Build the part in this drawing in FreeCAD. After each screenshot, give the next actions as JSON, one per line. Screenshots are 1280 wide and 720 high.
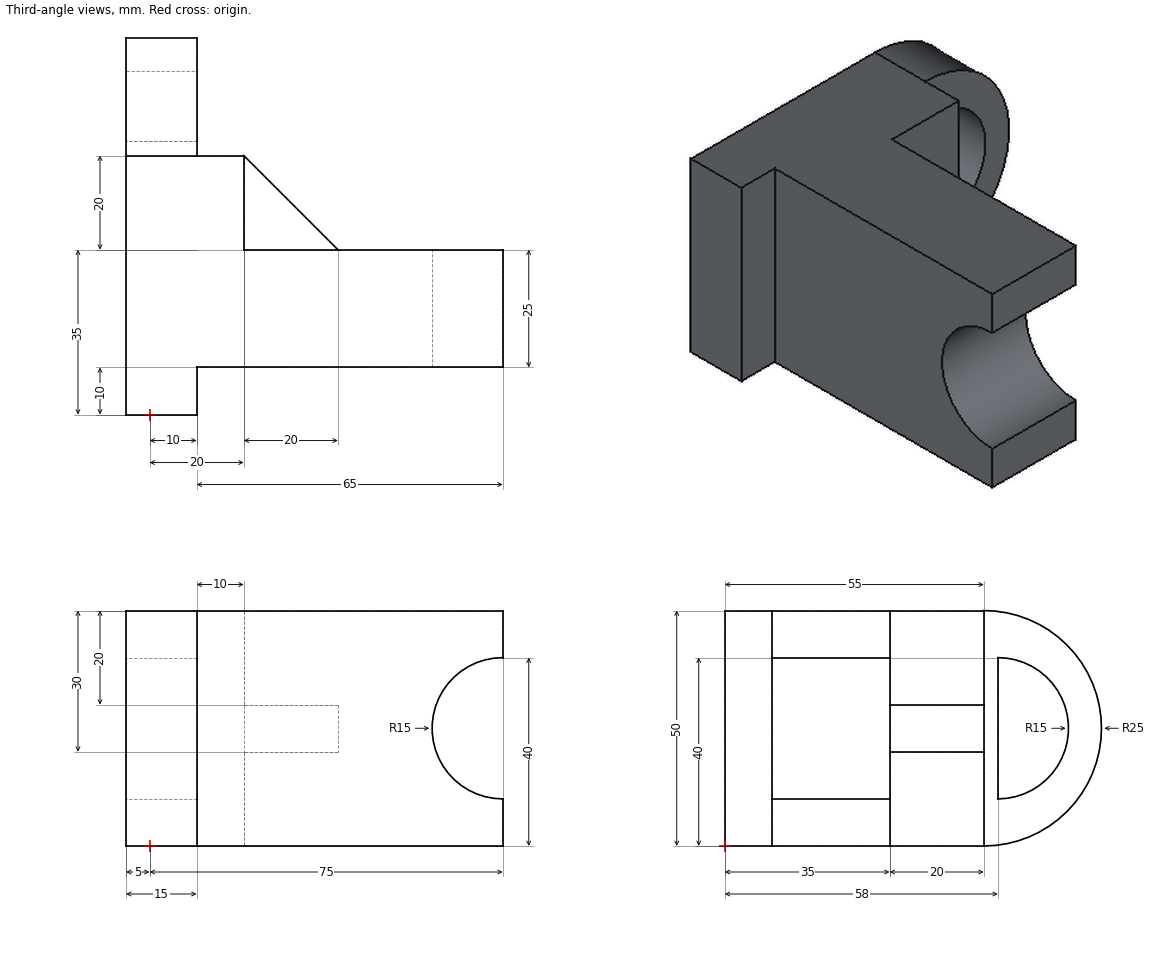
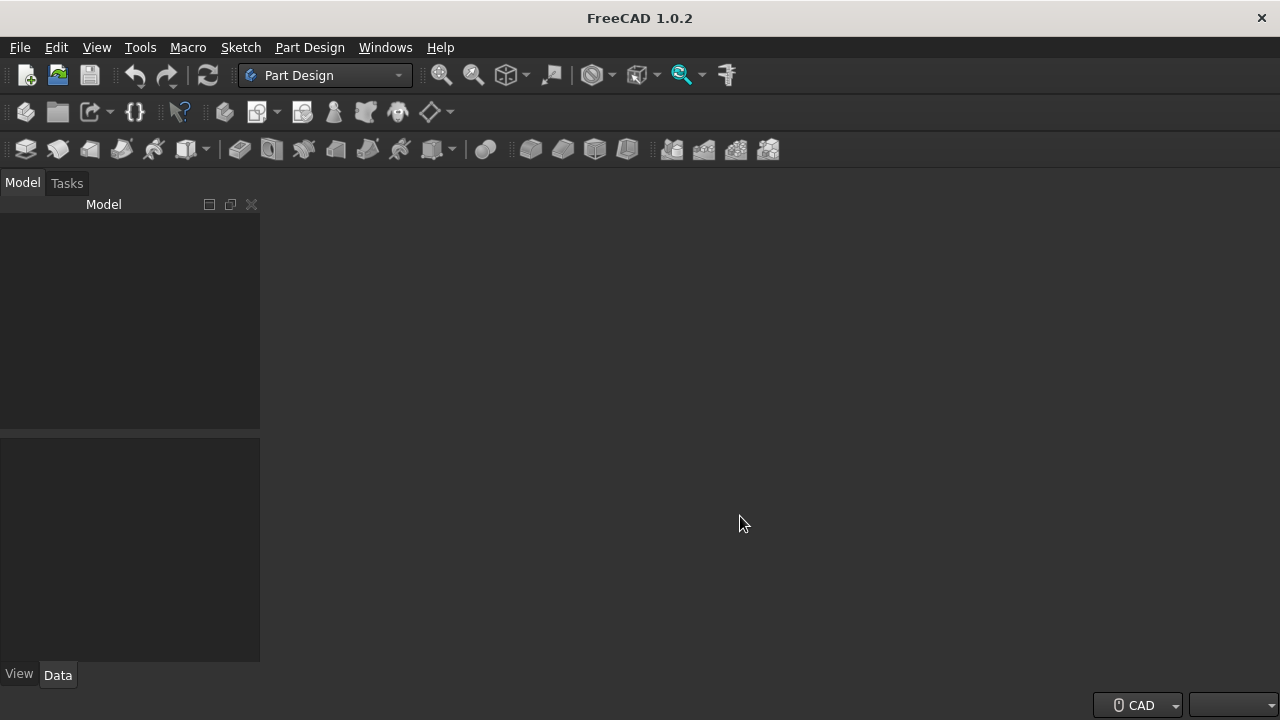
{"action": "left_click", "coordinate": [26, 76]}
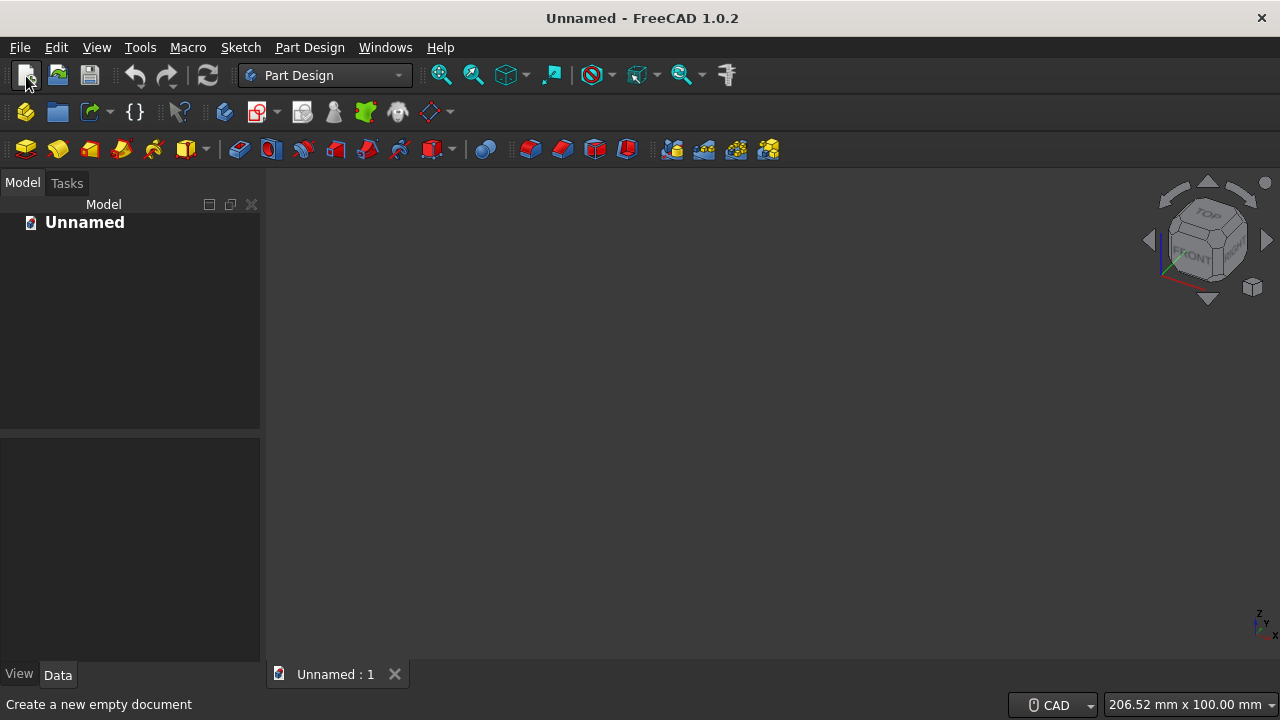
{"action": "left_click", "coordinate": [258, 112]}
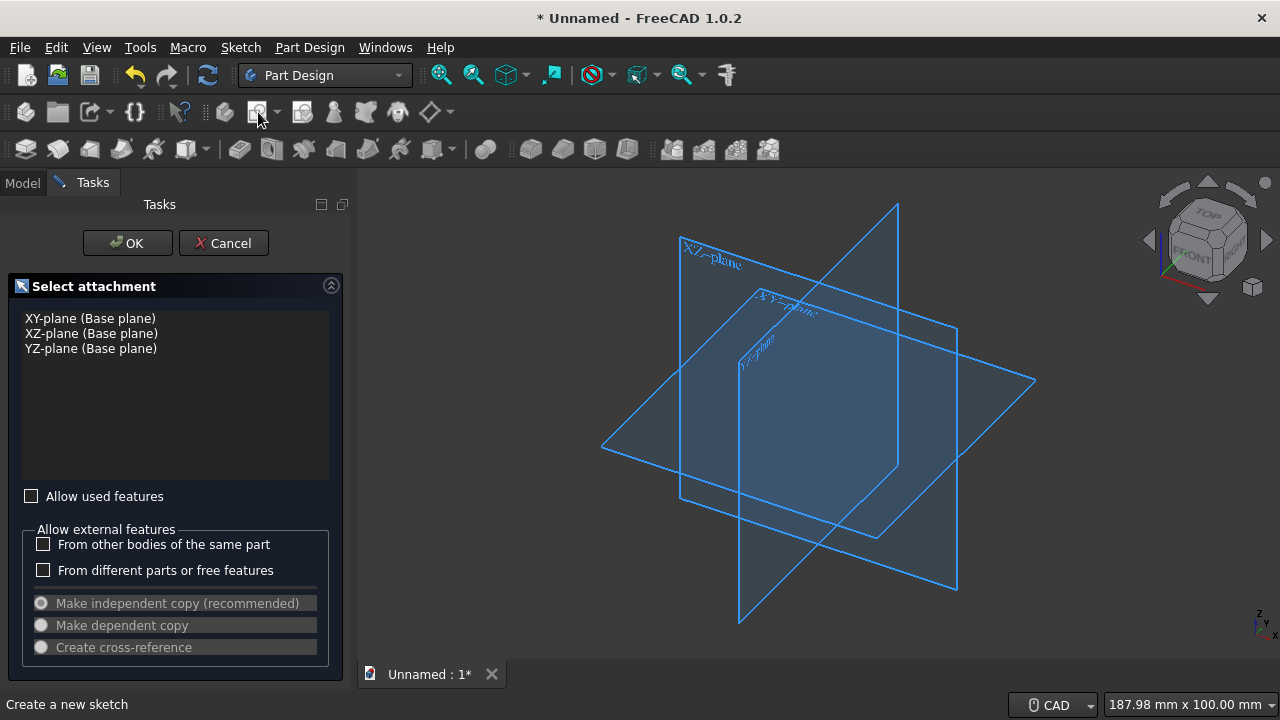
{"action": "left_click", "coordinate": [82, 318]}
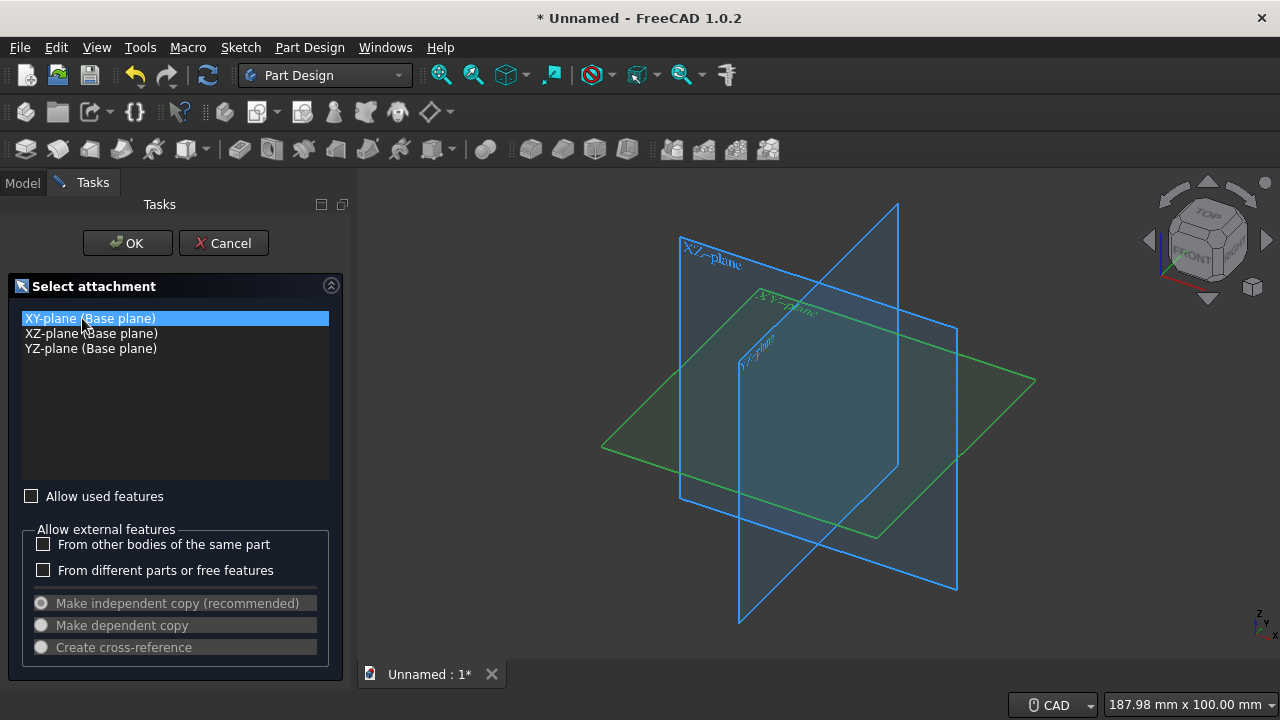
{"action": "left_click", "coordinate": [128, 243]}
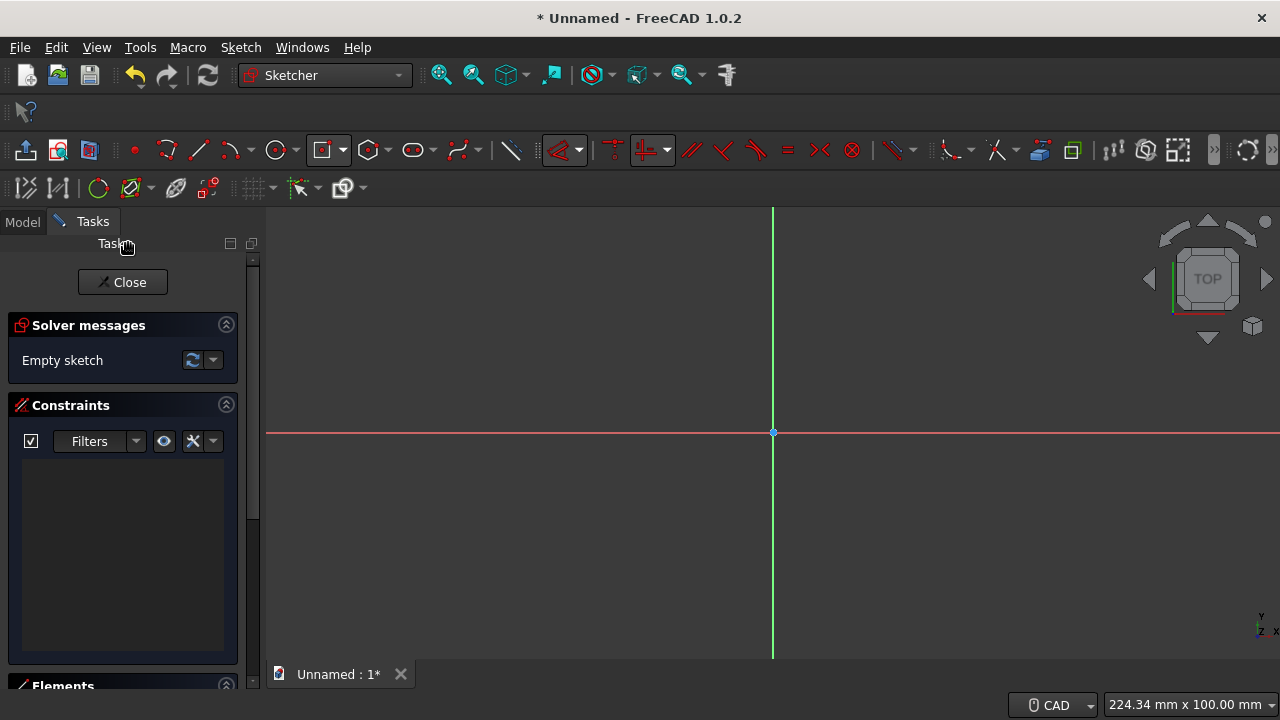
{"action": "scroll", "coordinate": [294, 631], "scroll_direction": "down", "scroll_amount": 1}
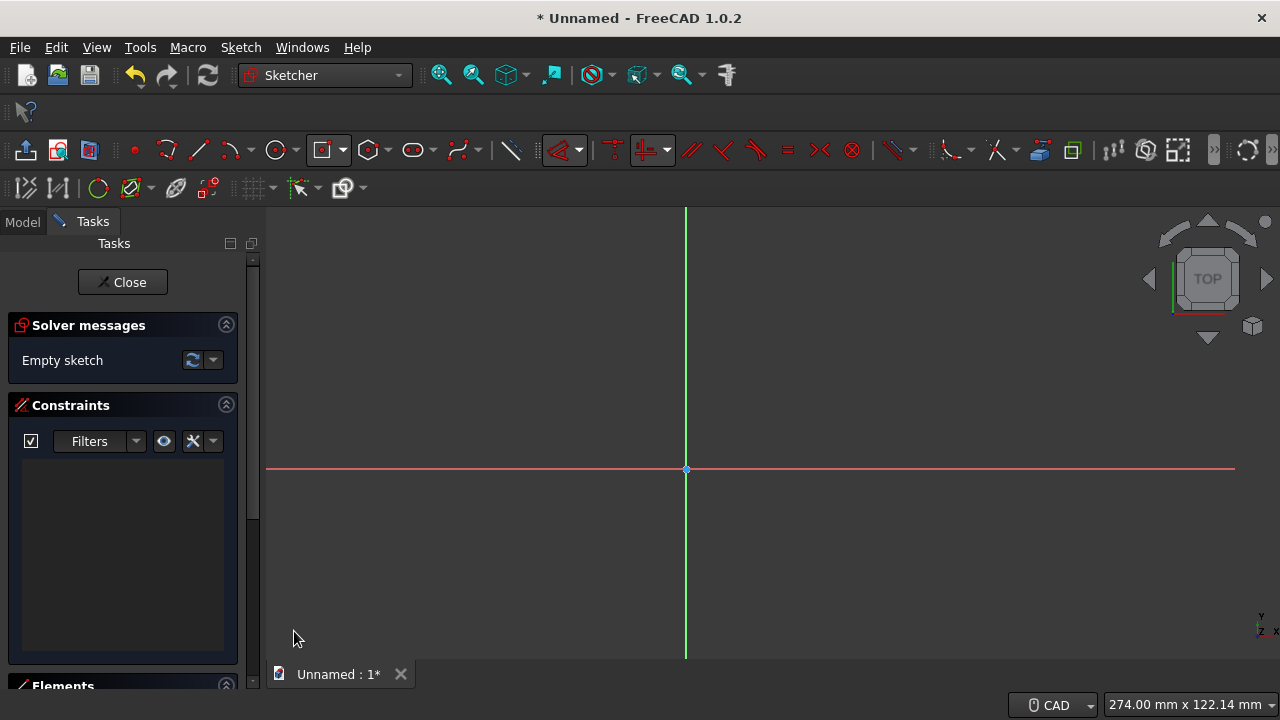
{"action": "scroll", "coordinate": [1070, 235], "scroll_direction": "up", "scroll_amount": 2}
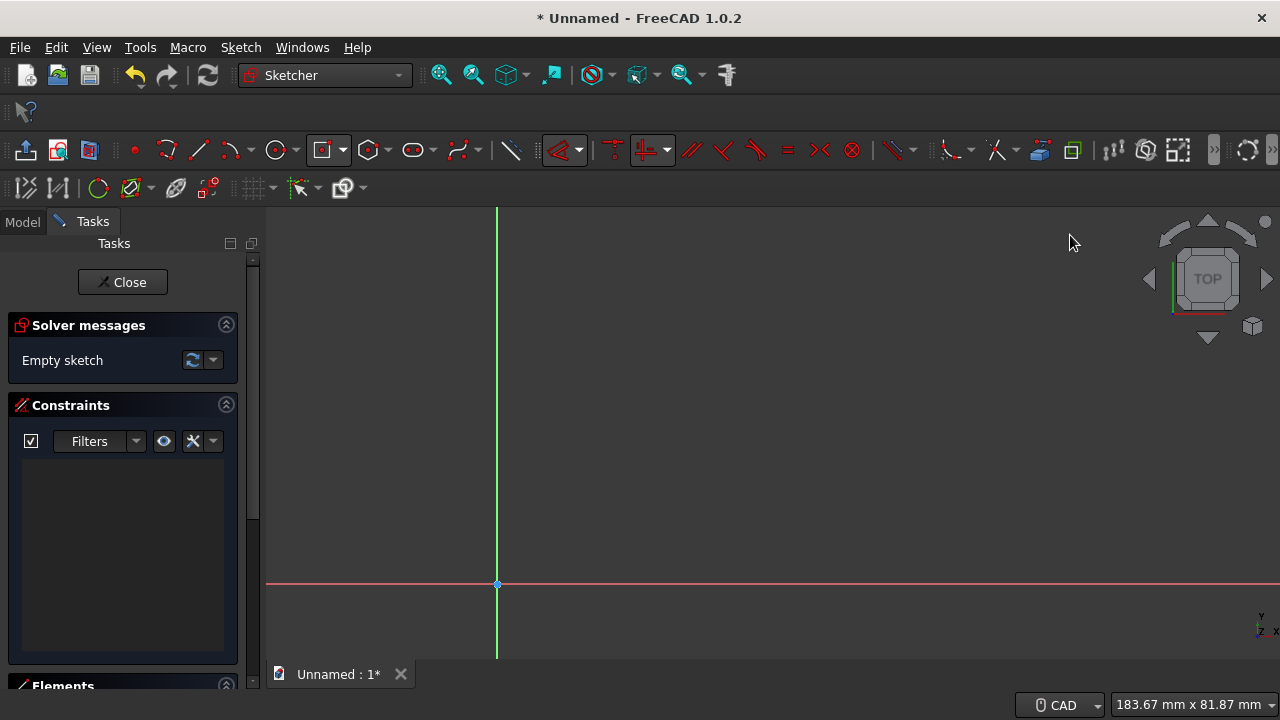
{"action": "left_click", "coordinate": [168, 150]}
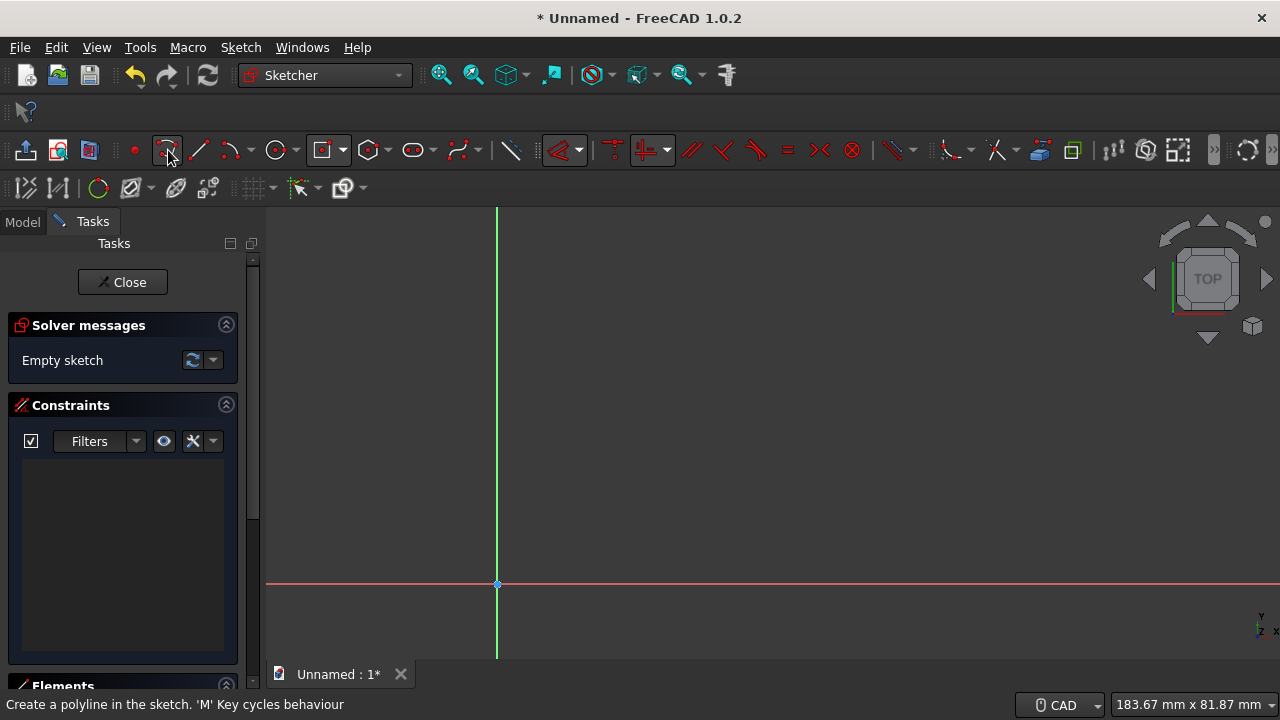
{"action": "left_click", "coordinate": [497, 584]}
{"action": "left_click", "coordinate": [552, 575]}
{"action": "left_click", "coordinate": [552, 529]}
{"action": "left_click", "coordinate": [911, 529]}
{"action": "left_click", "coordinate": [911, 391]}
{"action": "left_click", "coordinate": [552, 391]}
{"action": "left_click", "coordinate": [552, 281]}
{"action": "left_click", "coordinate": [506, 281]}
{"action": "left_click", "coordinate": [497, 584]}
{"action": "key", "text": "Escape"}
{"action": "key", "text": "Escape"}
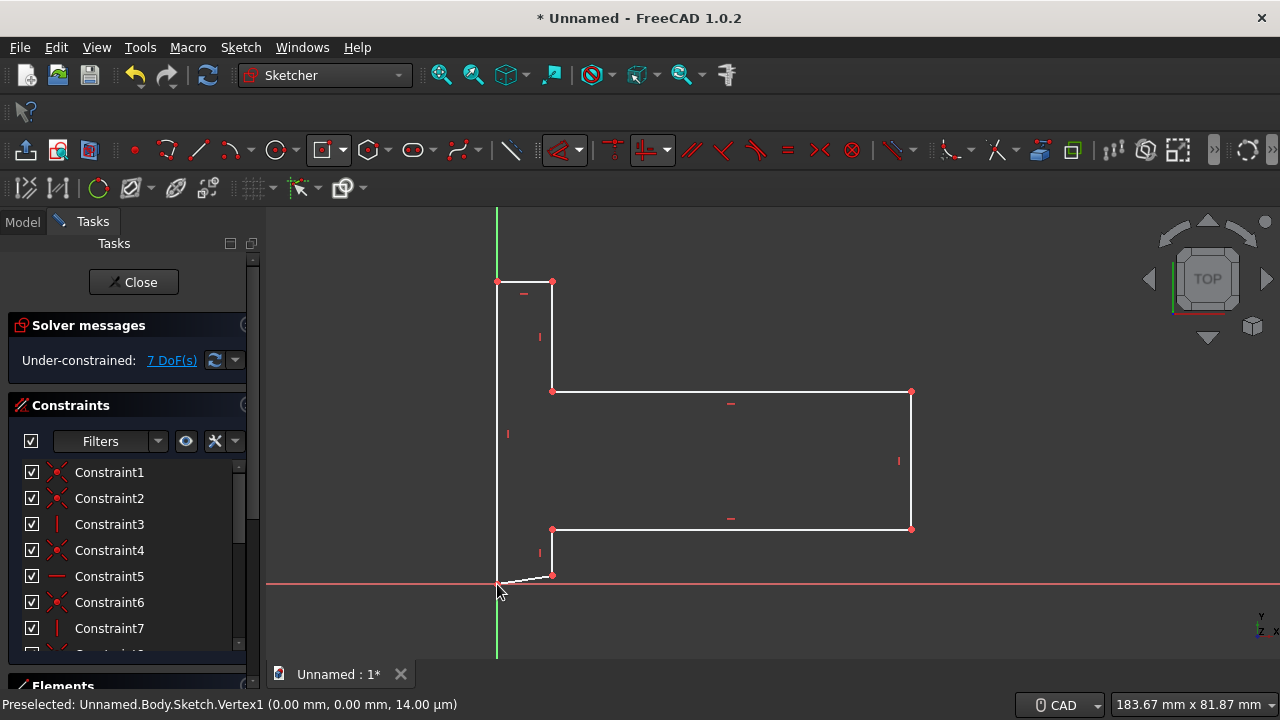
{"action": "left_click", "coordinate": [514, 582]}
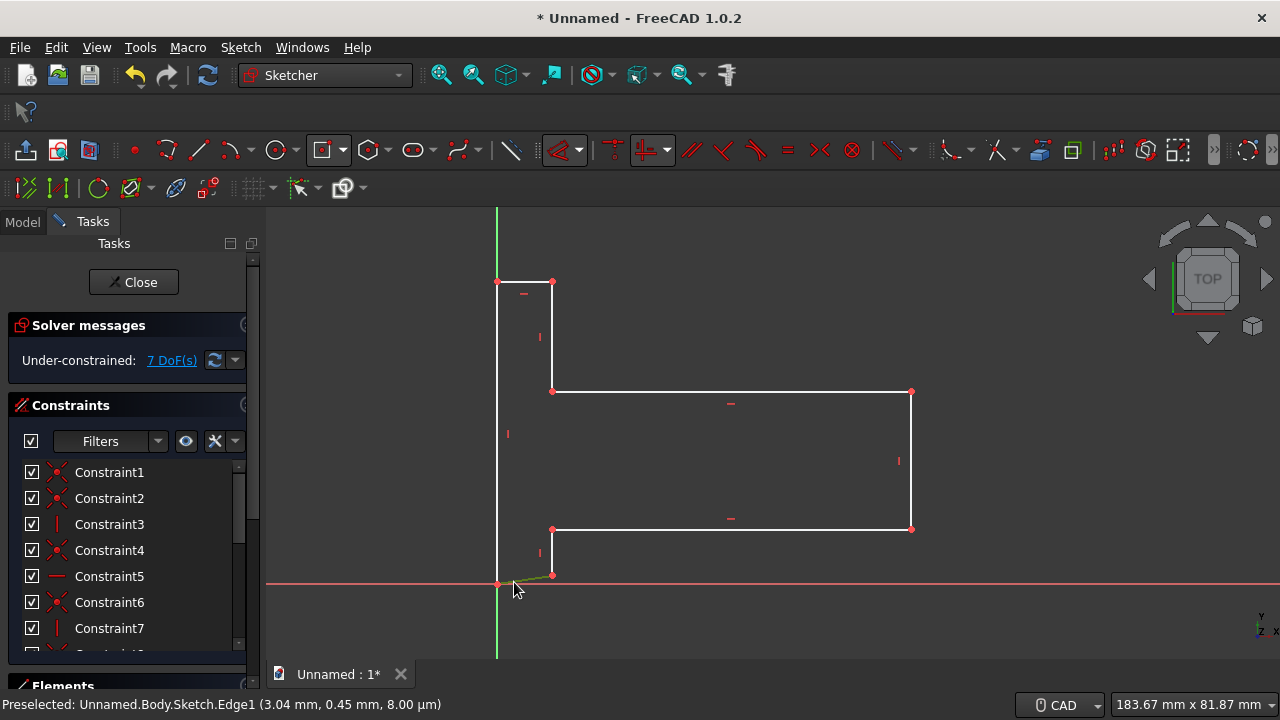
{"action": "left_click", "coordinate": [670, 150]}